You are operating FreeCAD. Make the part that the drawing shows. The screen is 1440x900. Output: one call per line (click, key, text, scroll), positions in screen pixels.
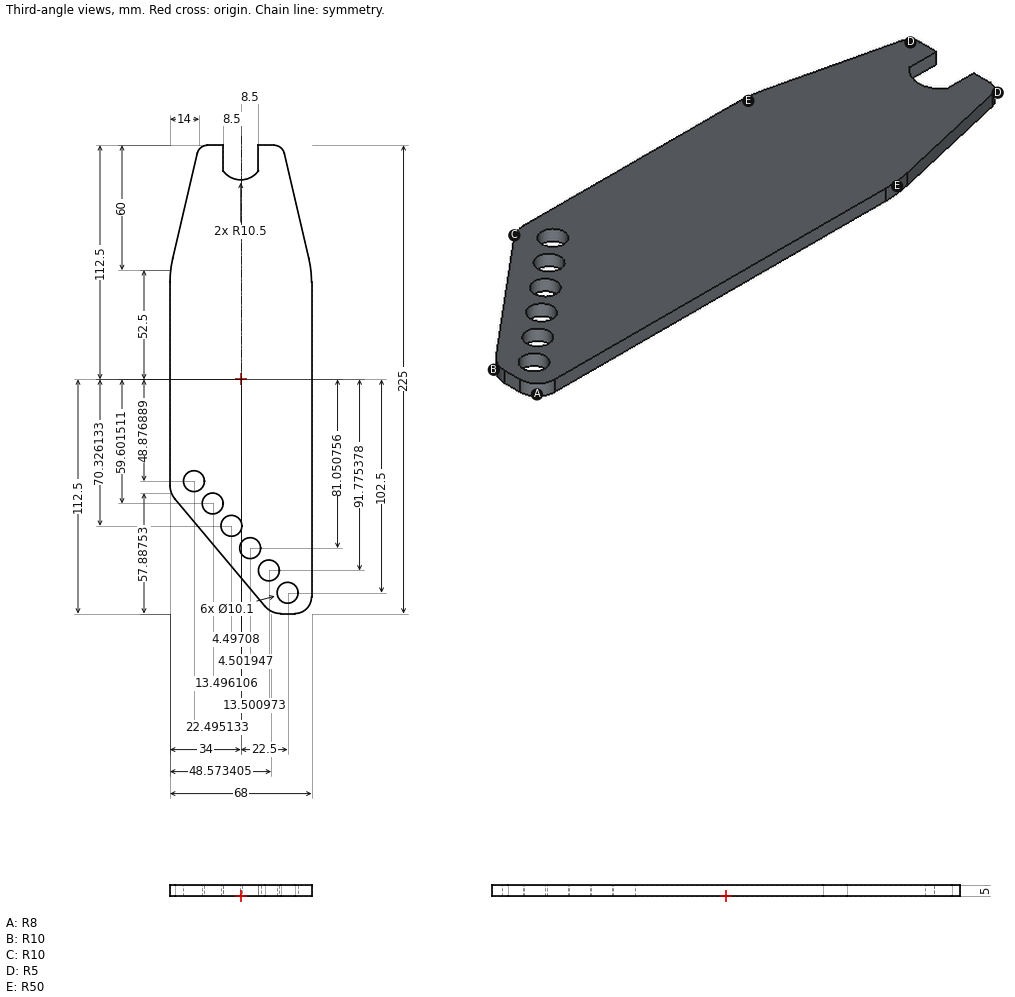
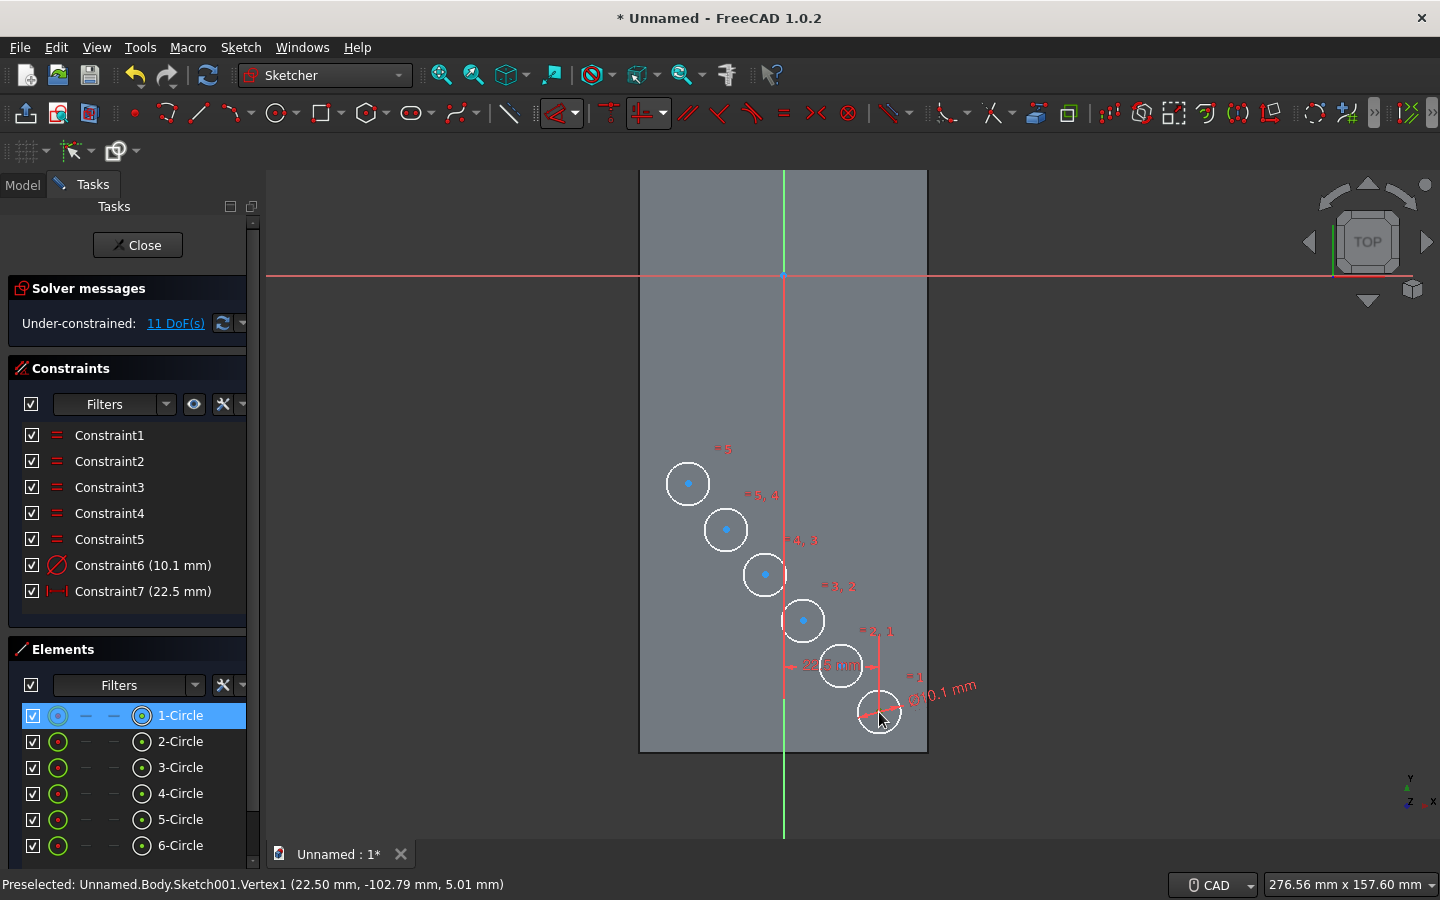
key(i)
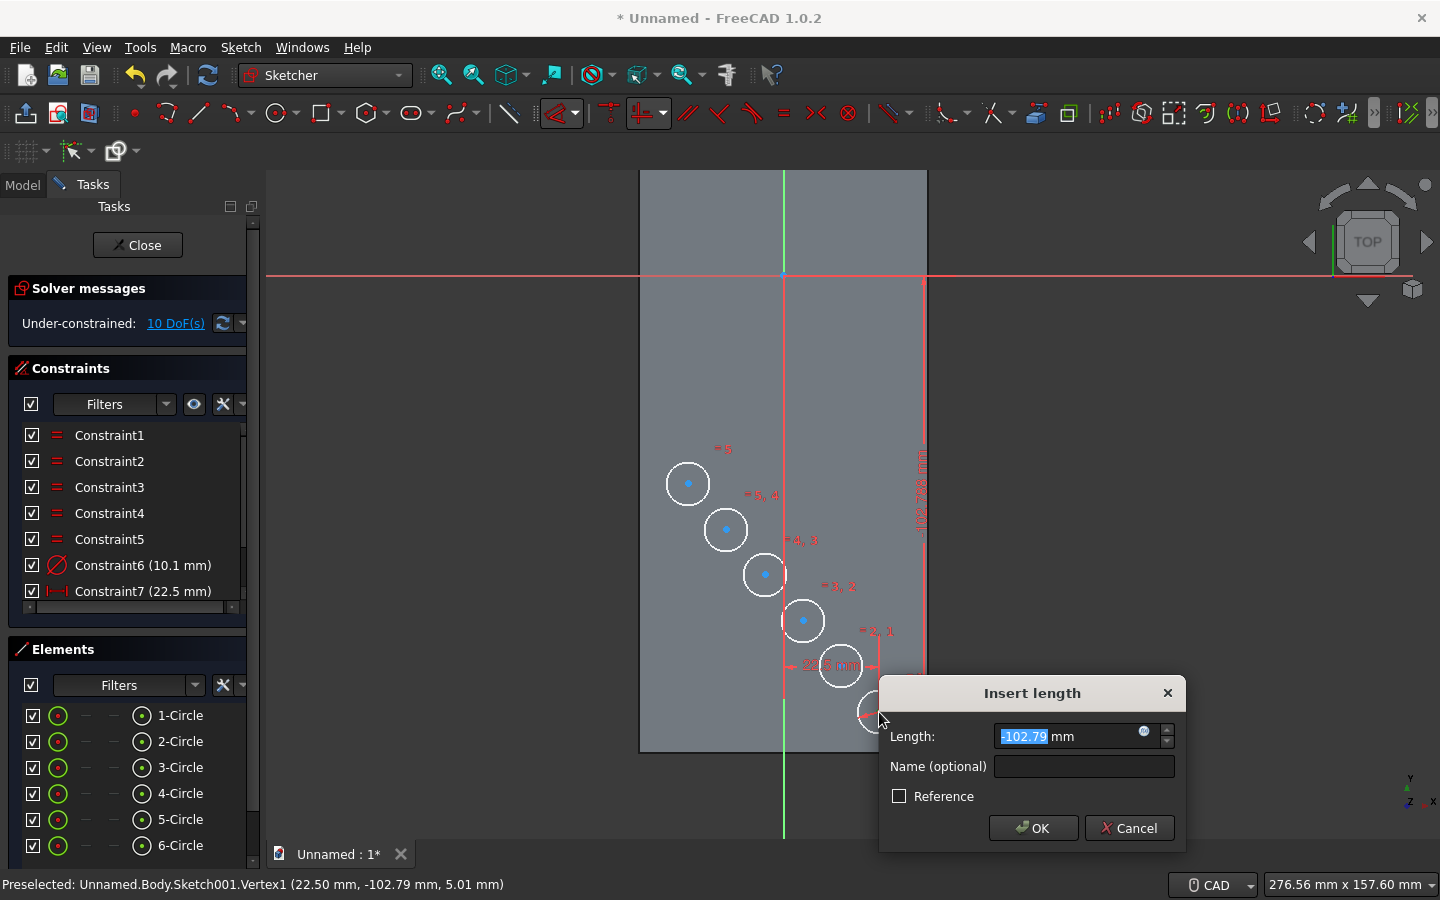
text(-102.5)
key(Return)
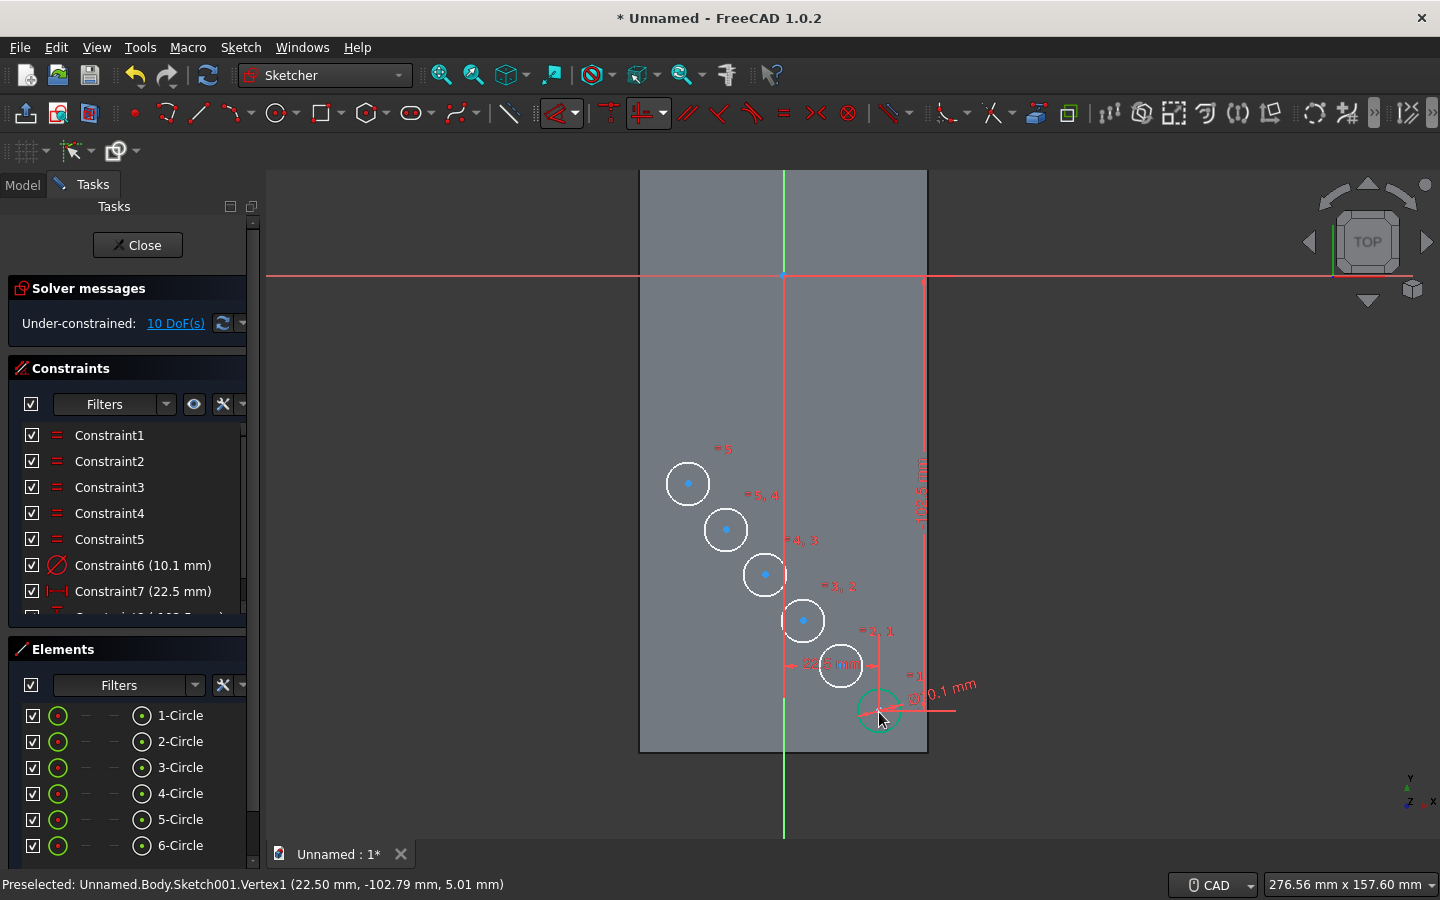
scroll(765, 575, up, 4)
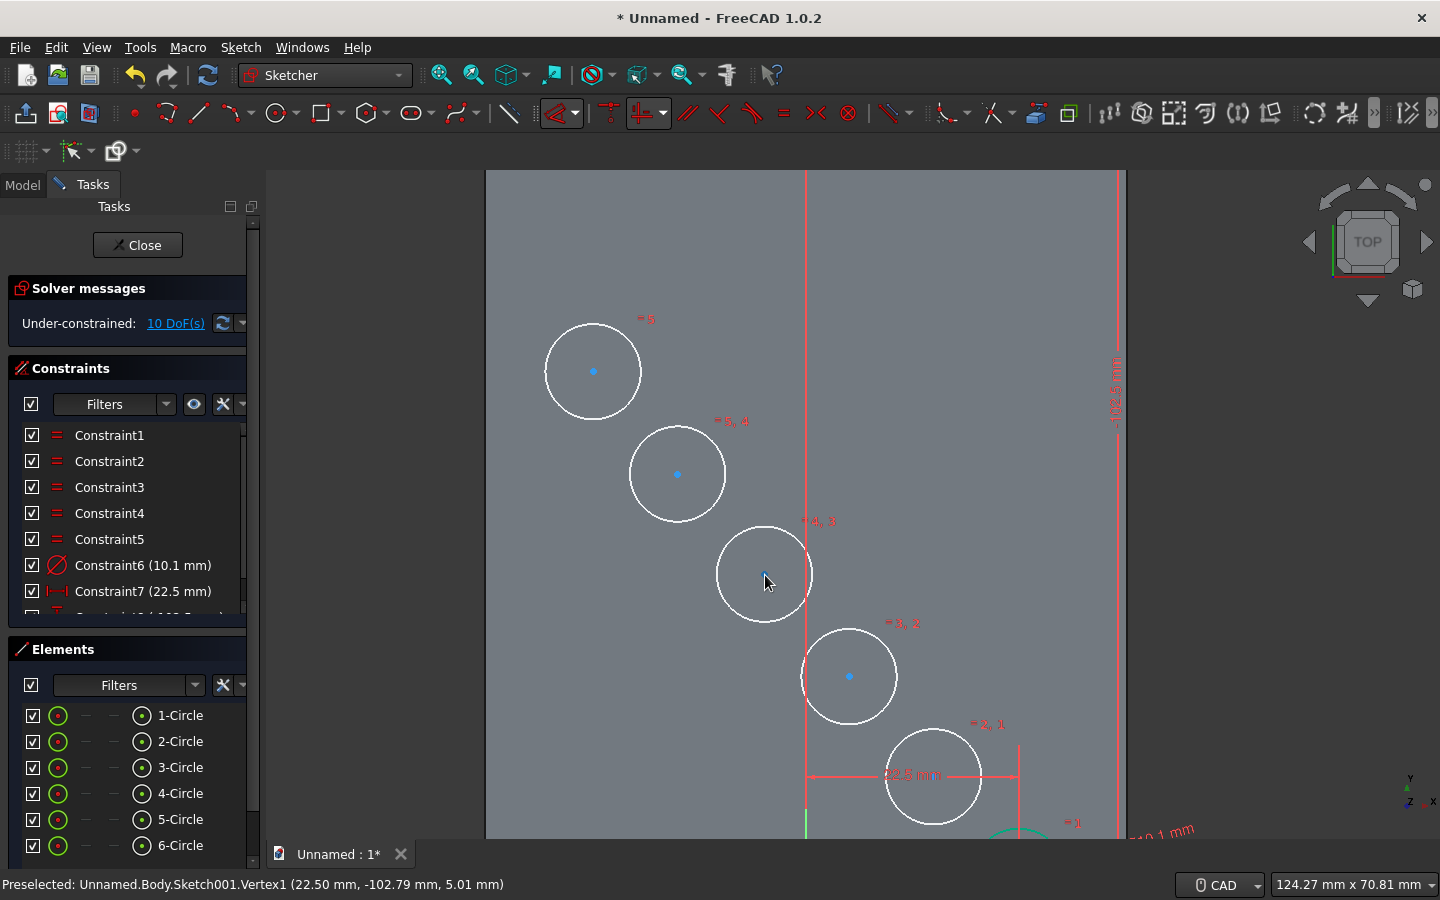
click(764, 574)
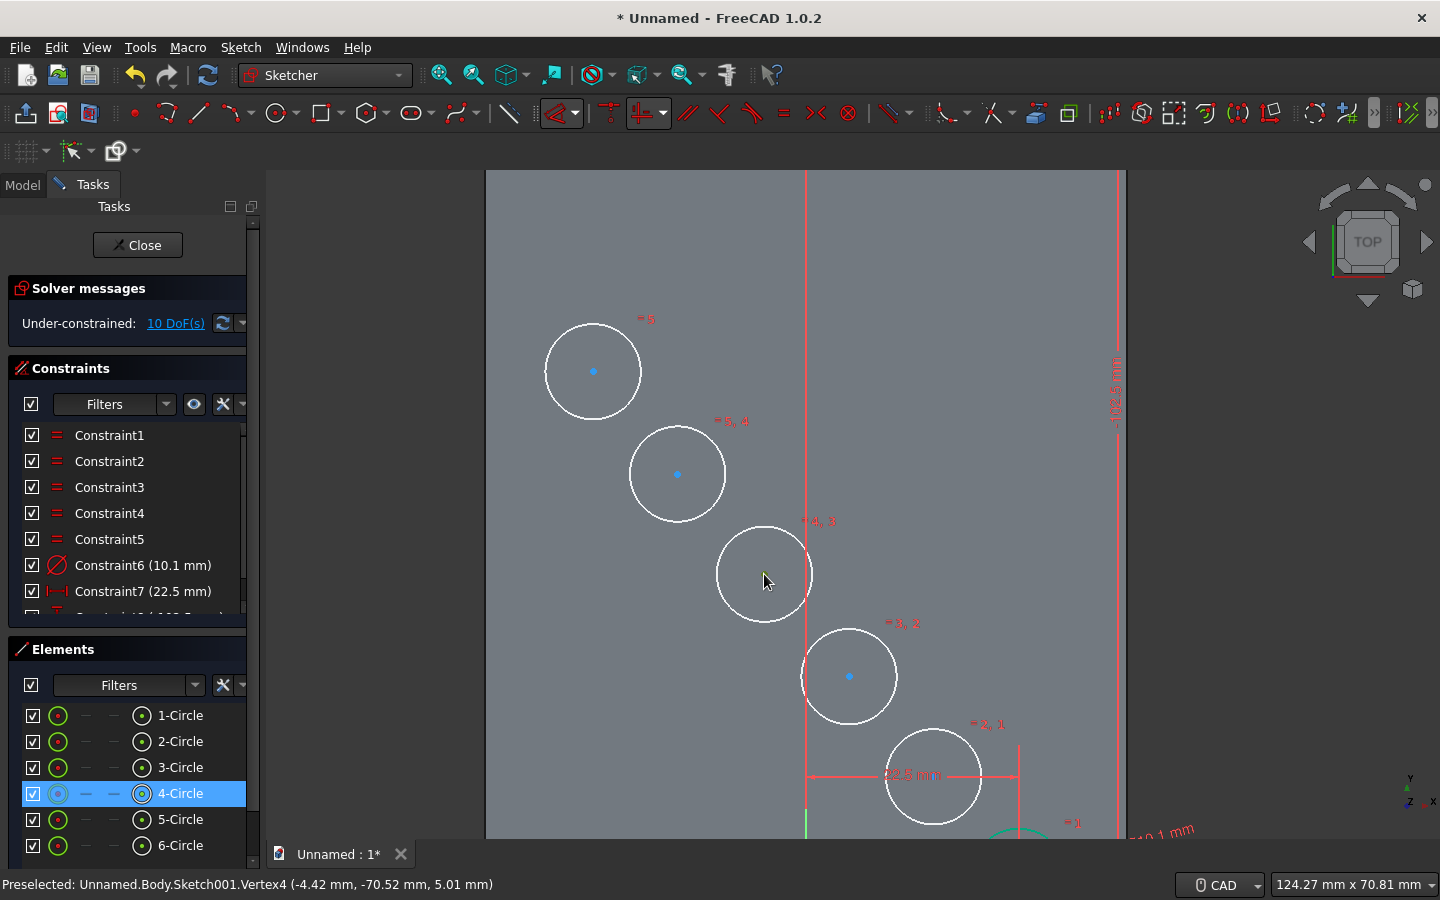
key(l)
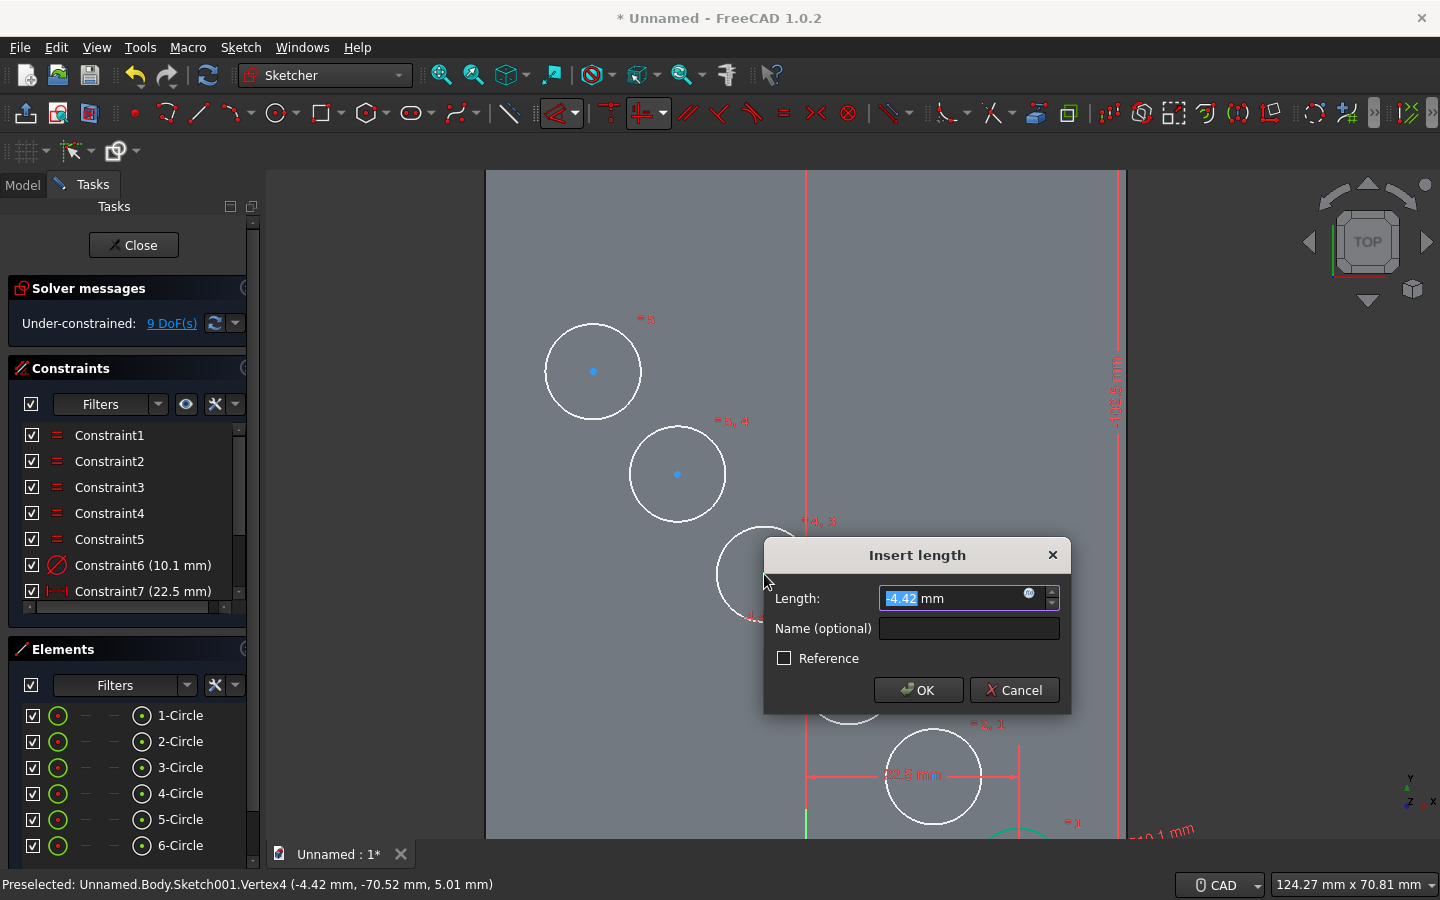
text(-4.49708)
key(Return)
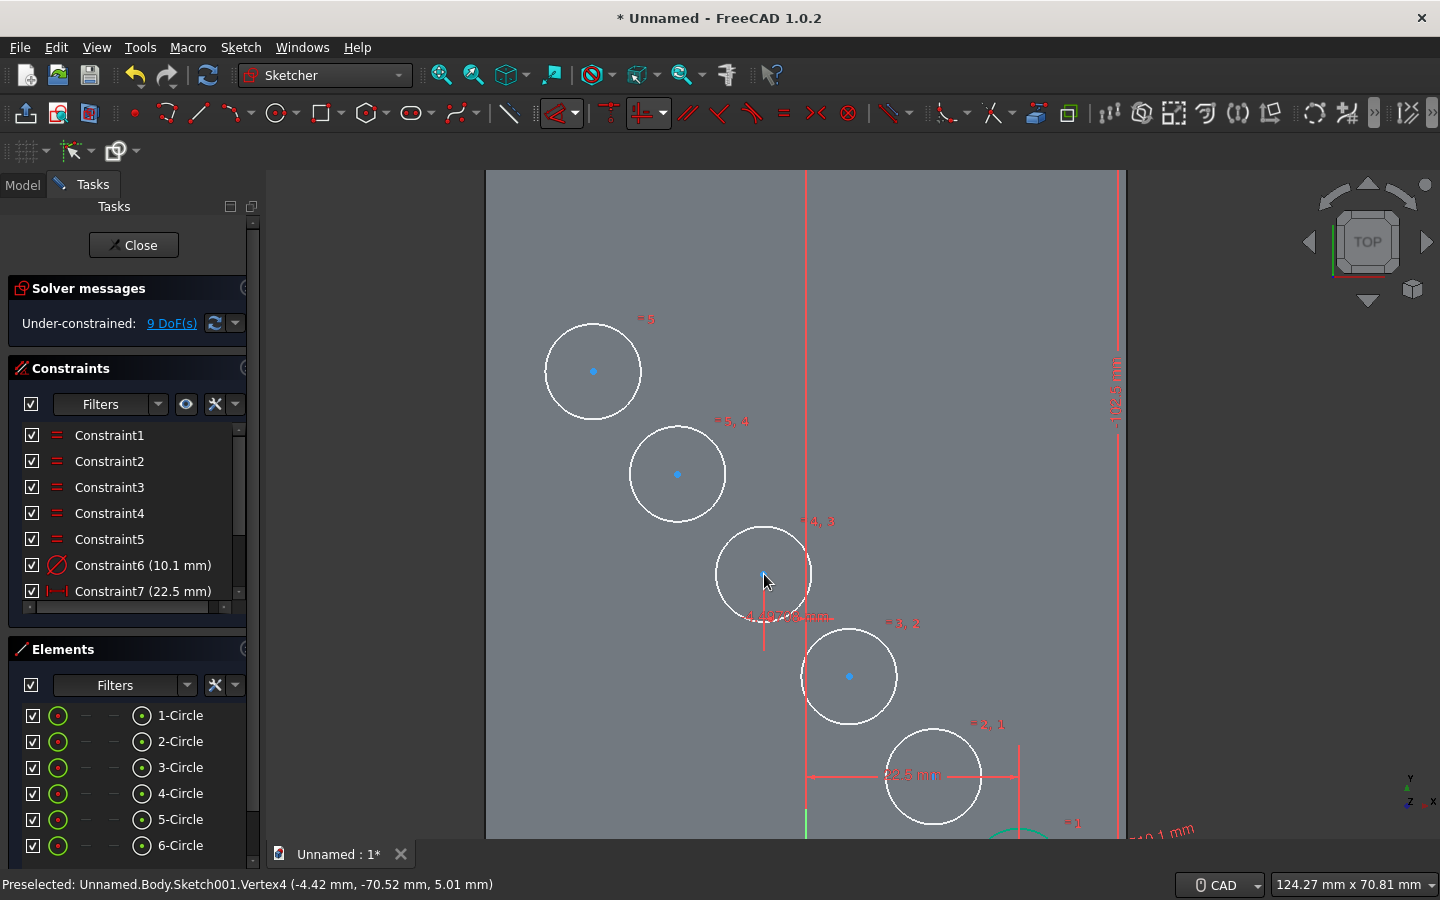
click(849, 677)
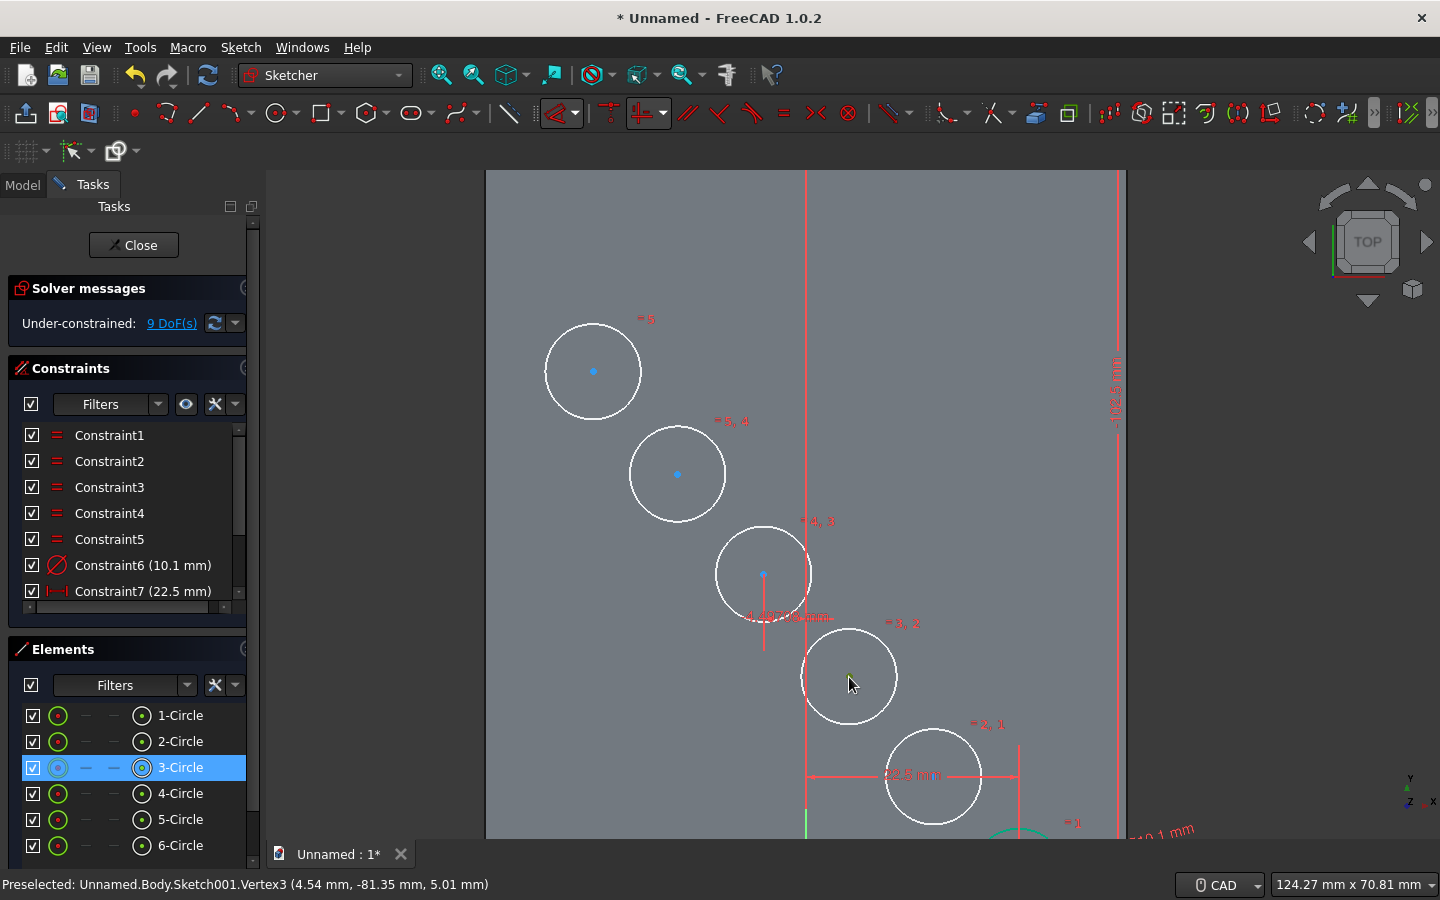
key(l)